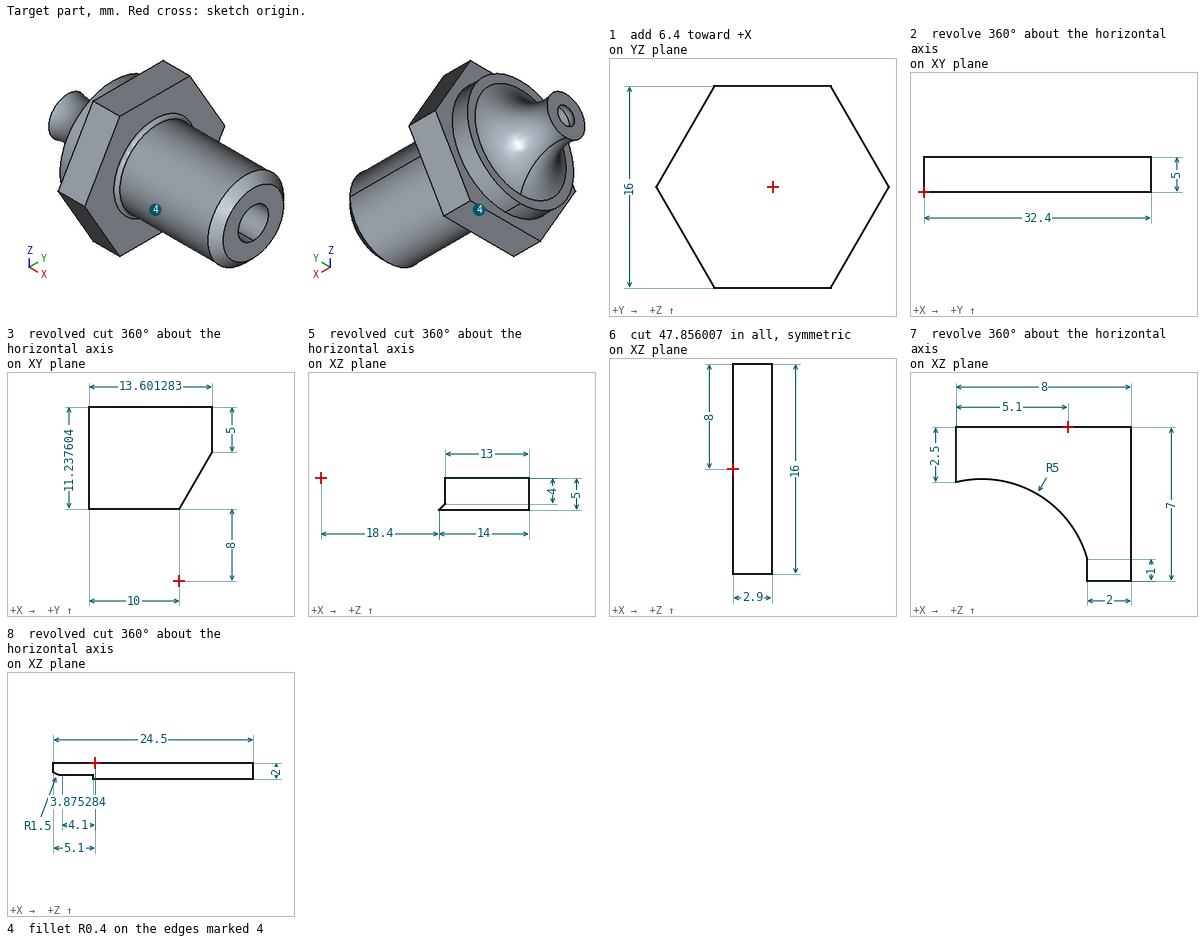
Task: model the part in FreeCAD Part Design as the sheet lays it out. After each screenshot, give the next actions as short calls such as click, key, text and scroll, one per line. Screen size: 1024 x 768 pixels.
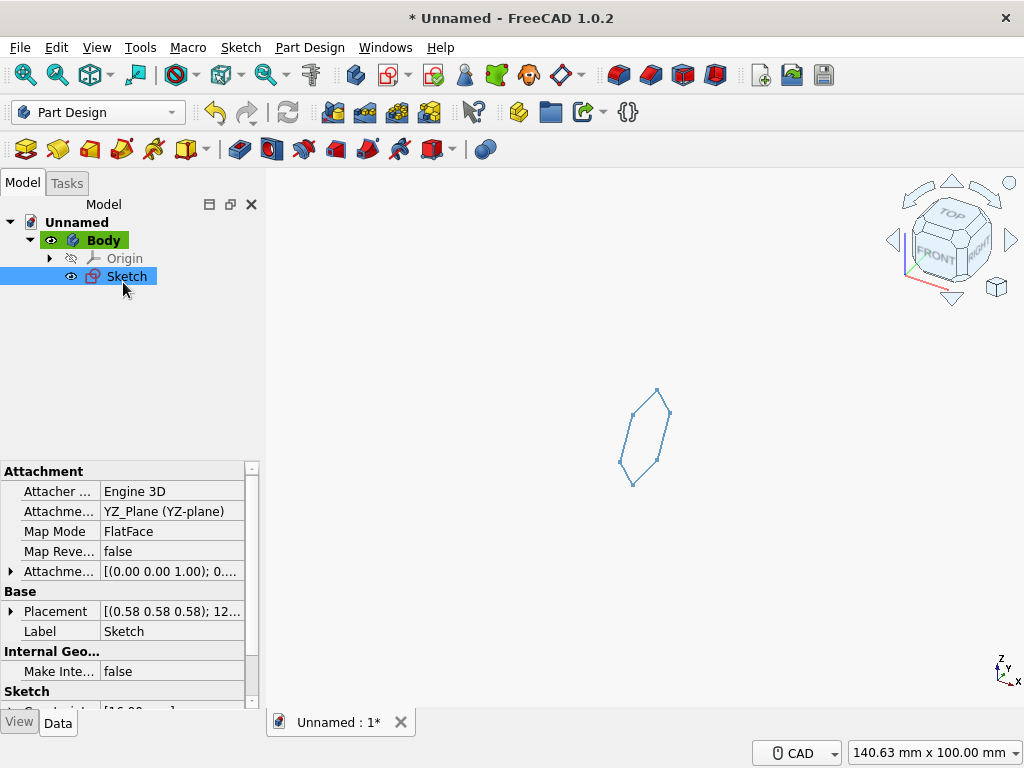
click(26, 150)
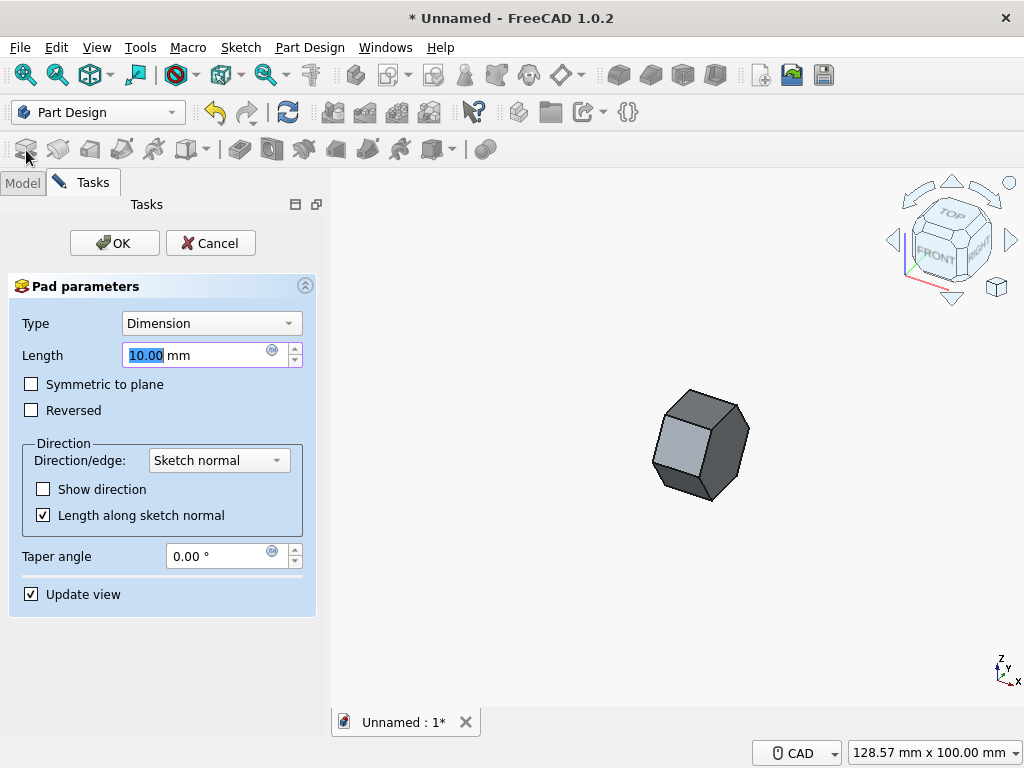
text(6.4)
key(Tab)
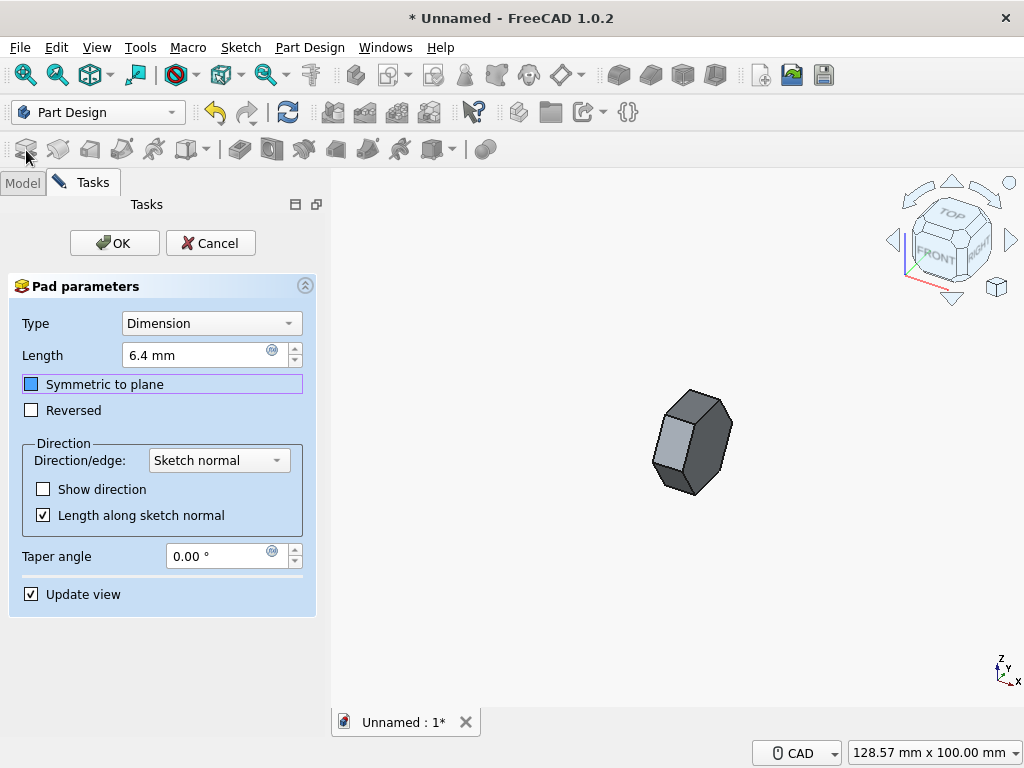
click(115, 243)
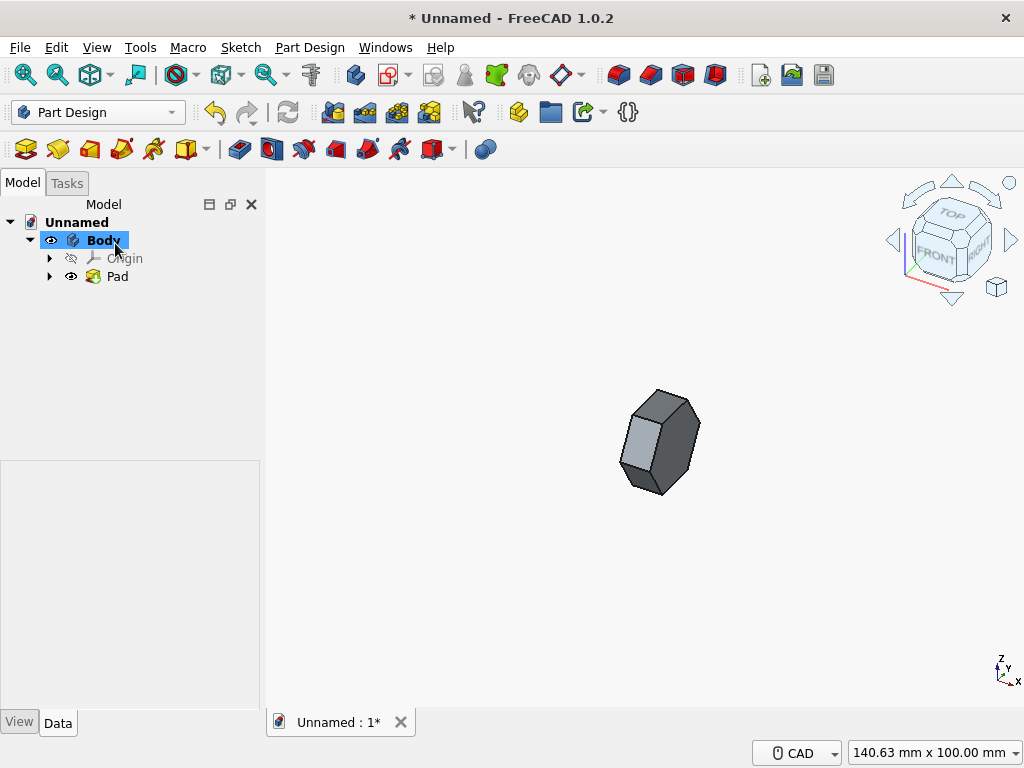
click(26, 76)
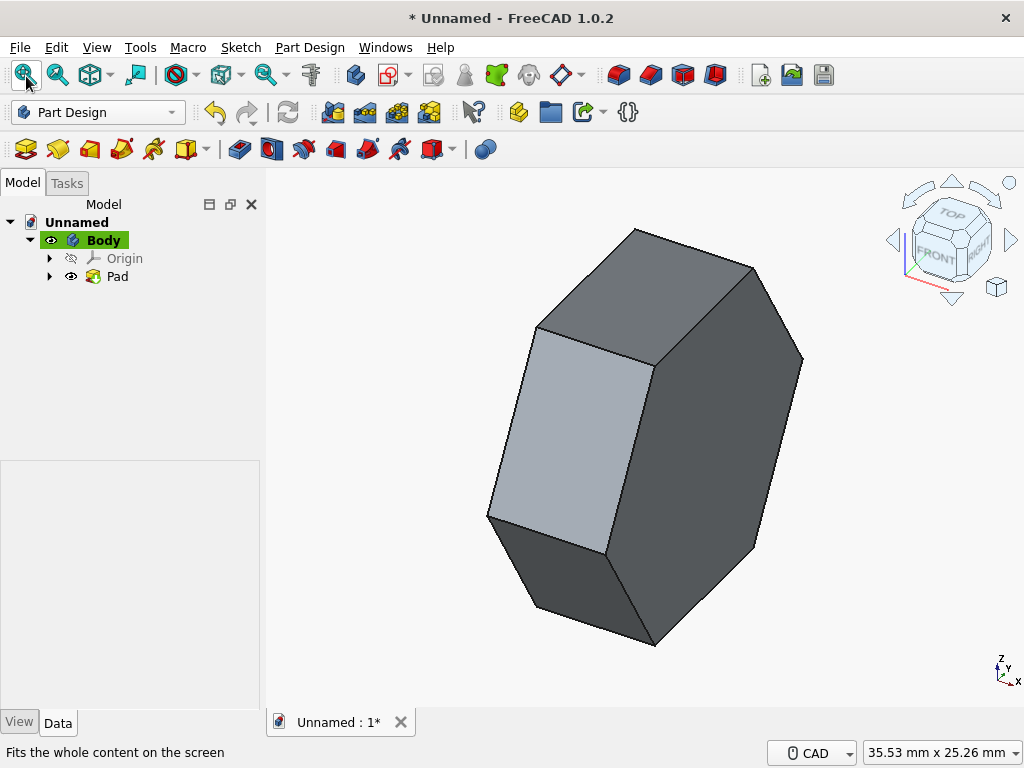
click(388, 76)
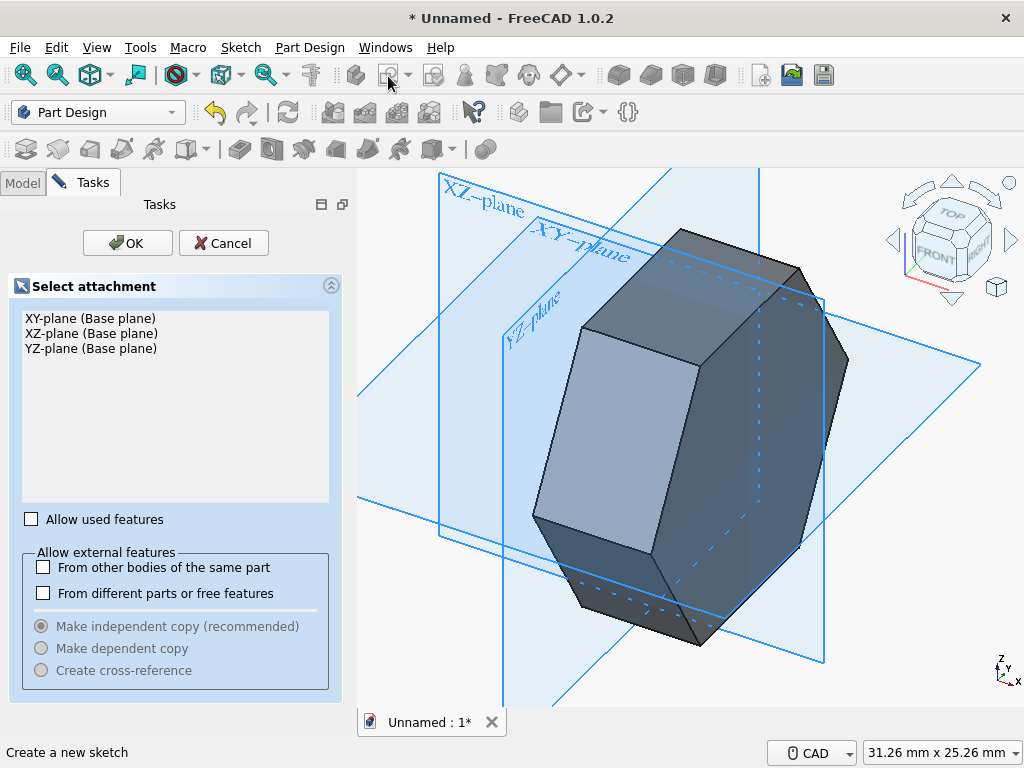
click(82, 318)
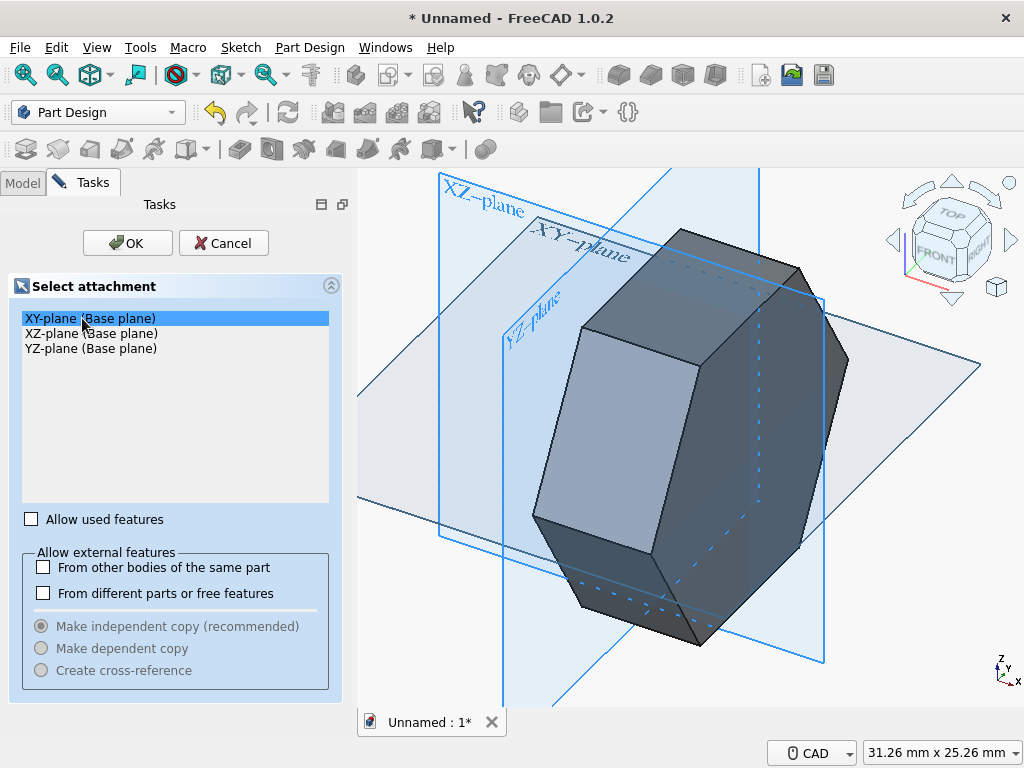
click(128, 243)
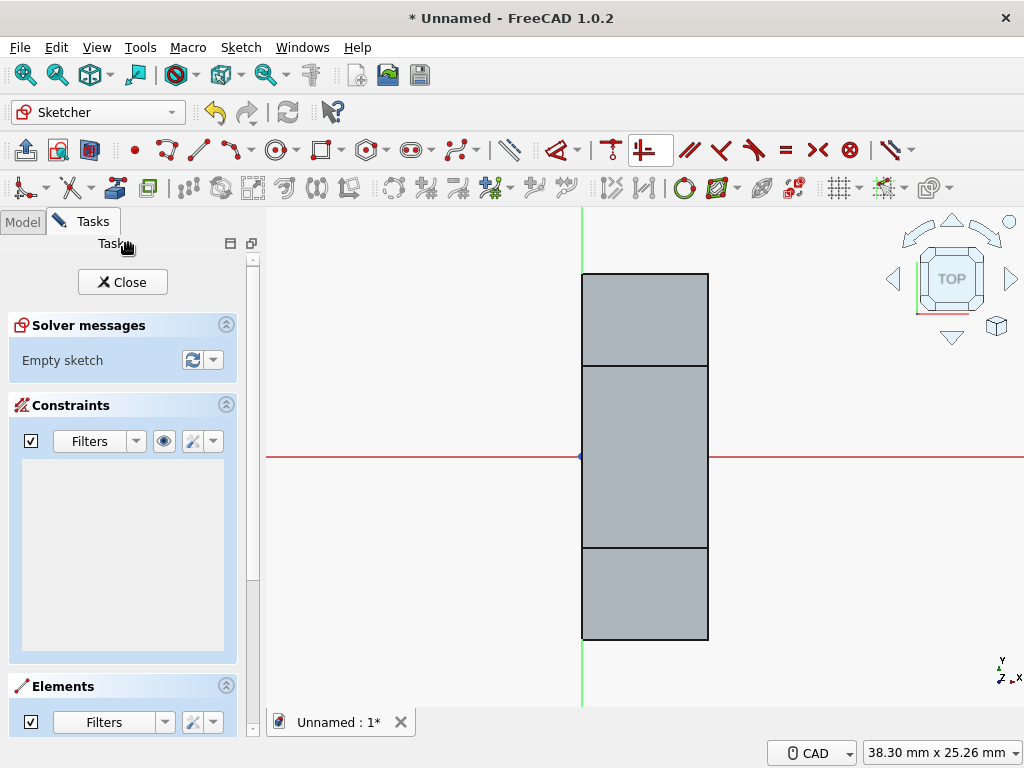
click(90, 150)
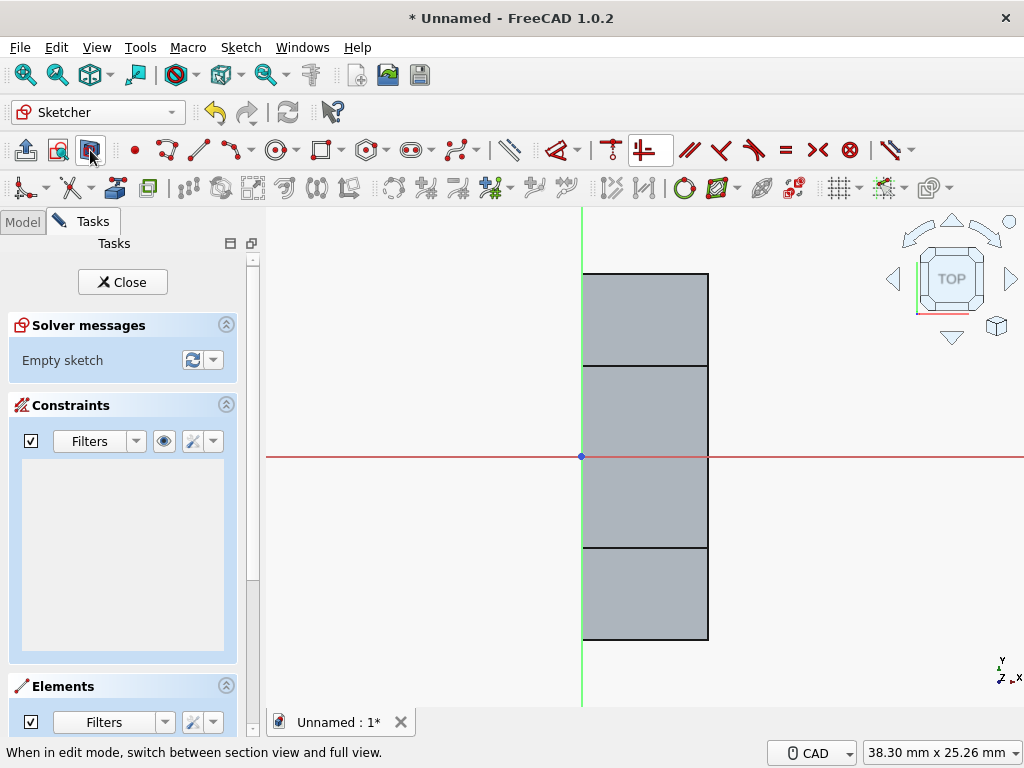
scroll(294, 517, down, 3)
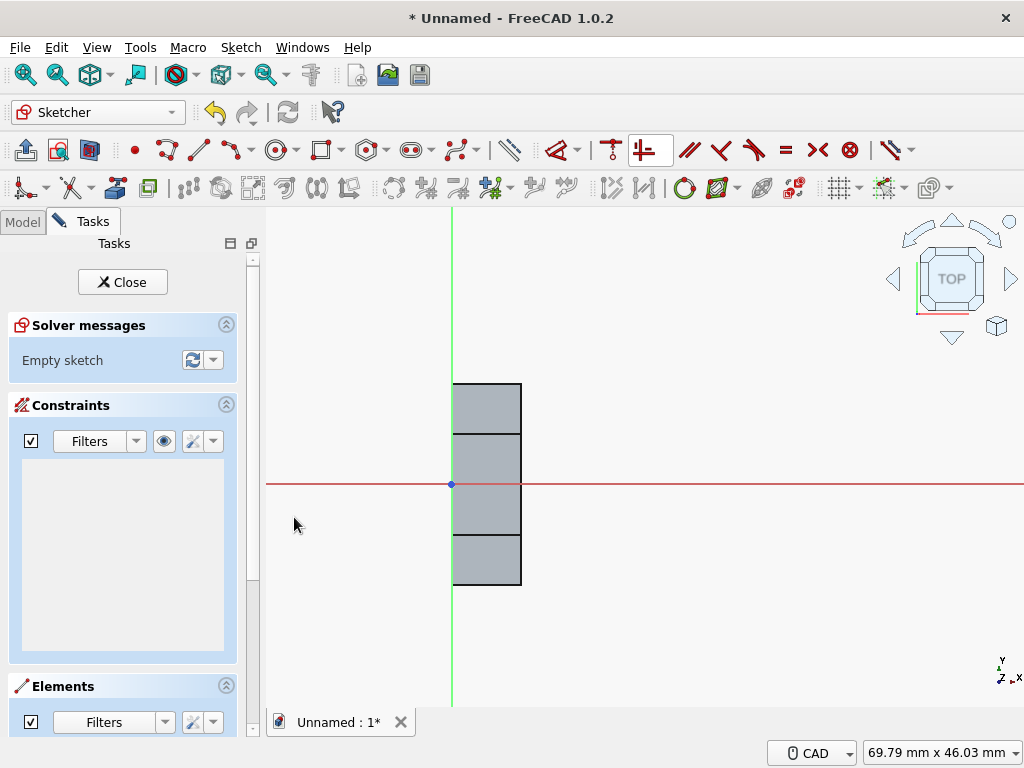
click(322, 150)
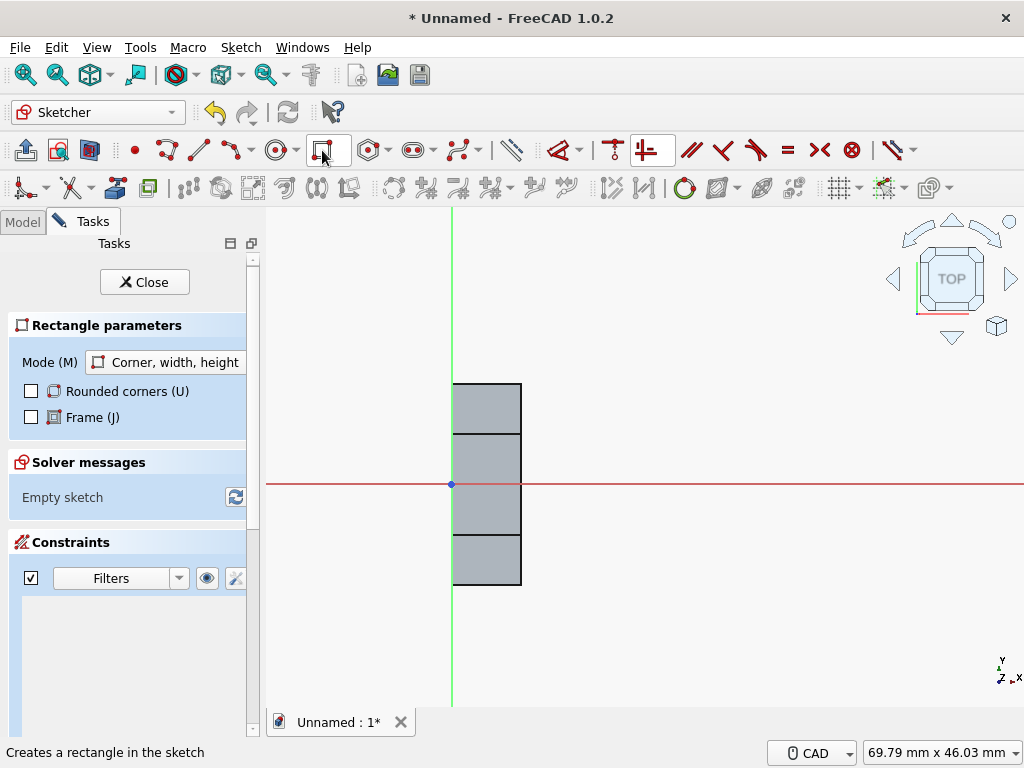
click(452, 484)
move(804, 430)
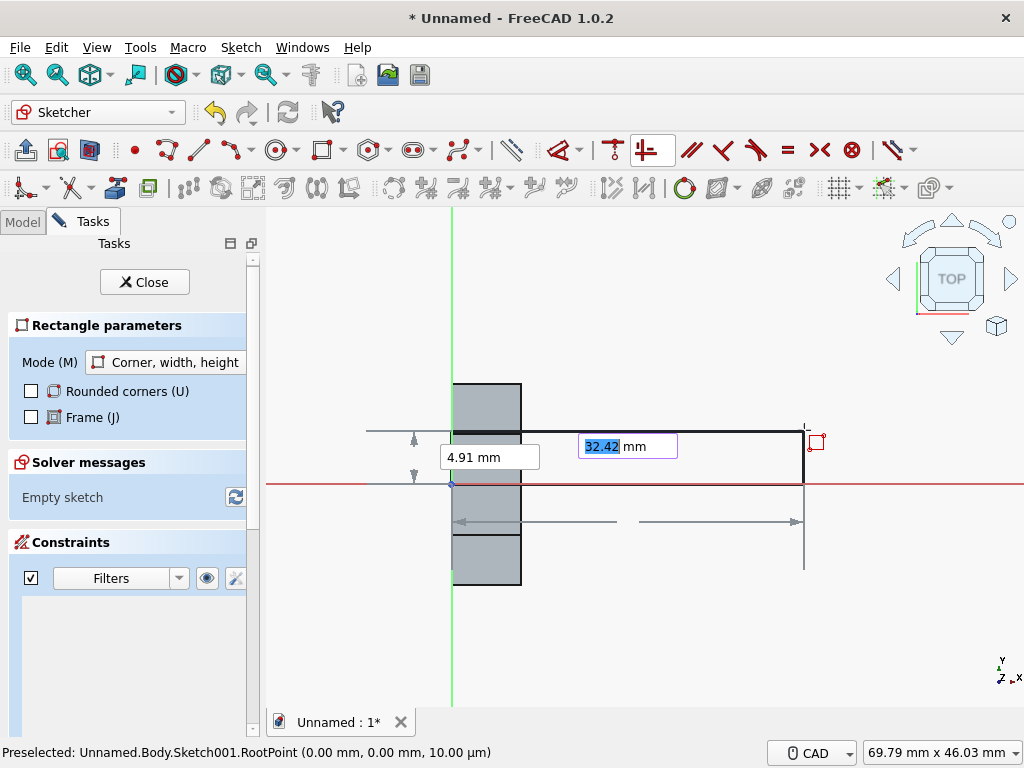
text(32.4)
key(Tab)
text(5)
key(Return)
key(Escape)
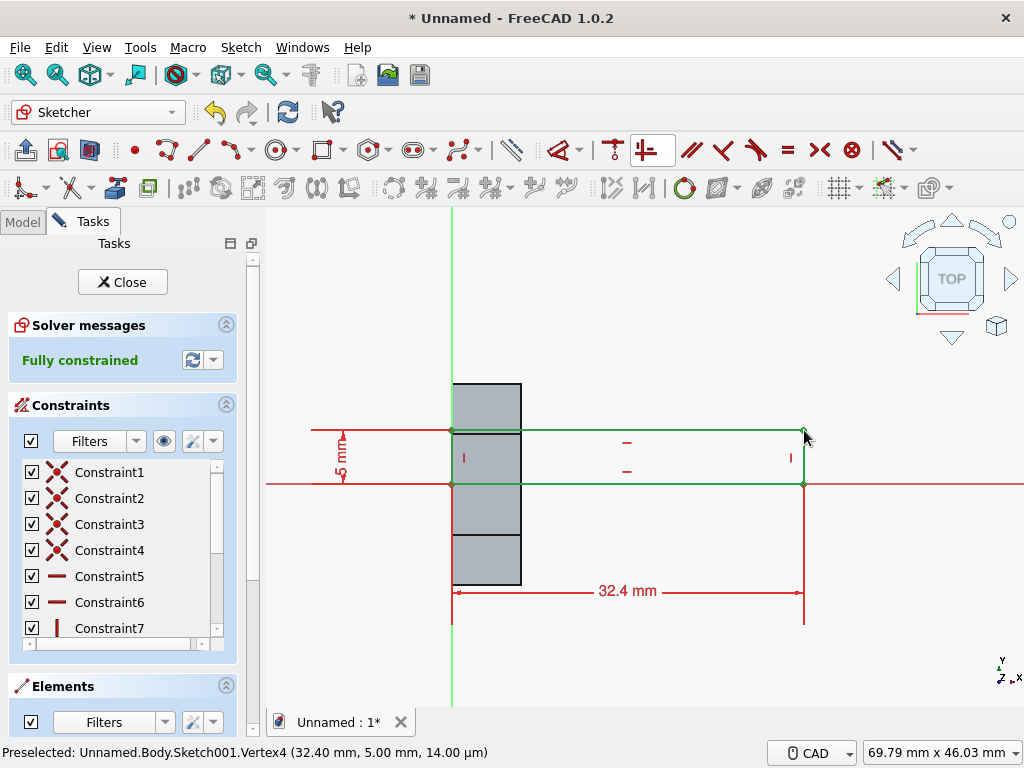
click(123, 282)